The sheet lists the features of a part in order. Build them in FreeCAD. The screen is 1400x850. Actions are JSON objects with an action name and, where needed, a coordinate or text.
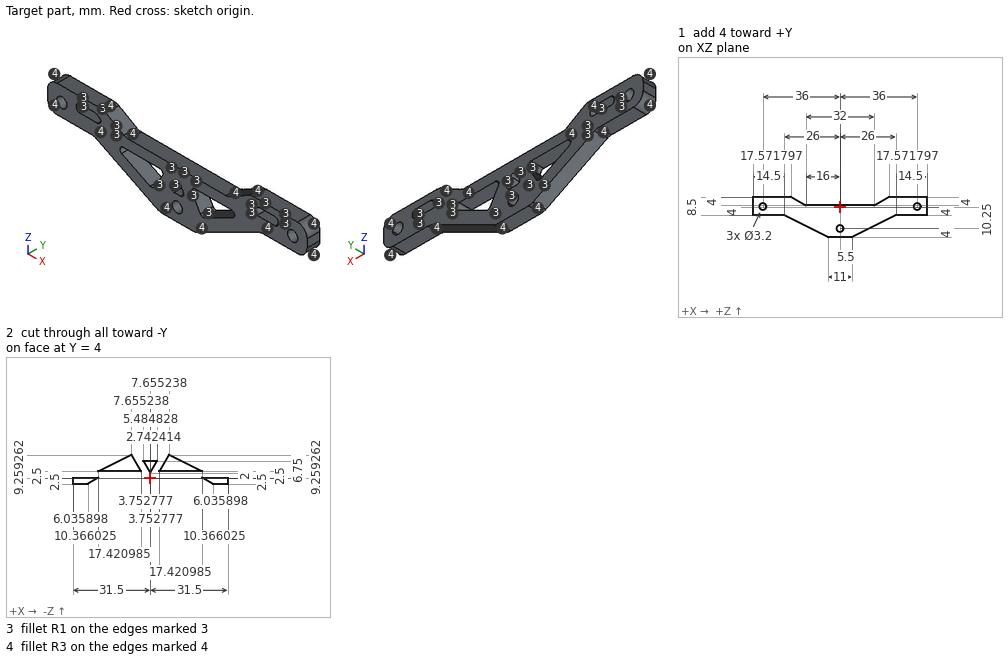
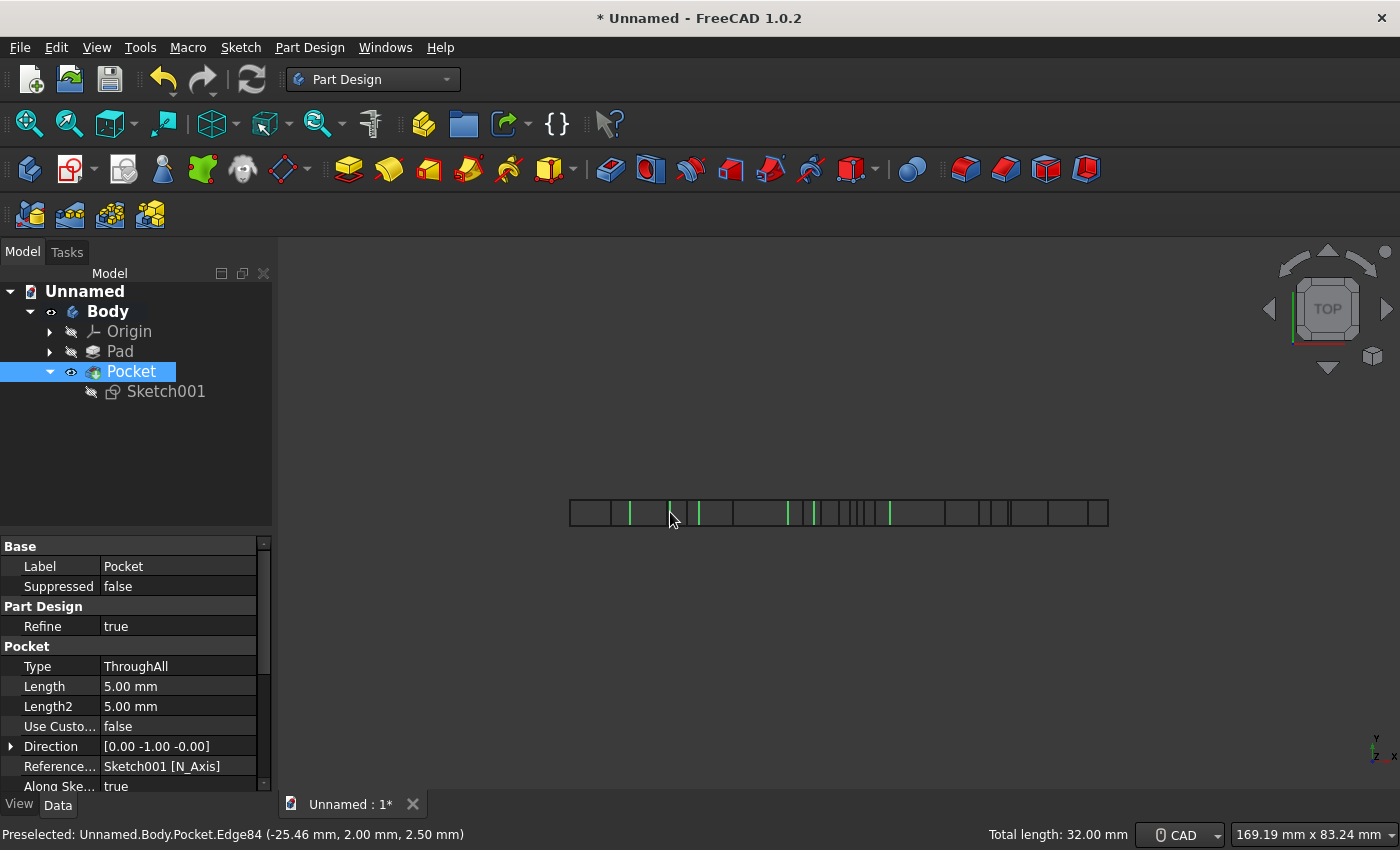
{"action": "left_click", "coordinate": [1008, 512], "text": "ctrl"}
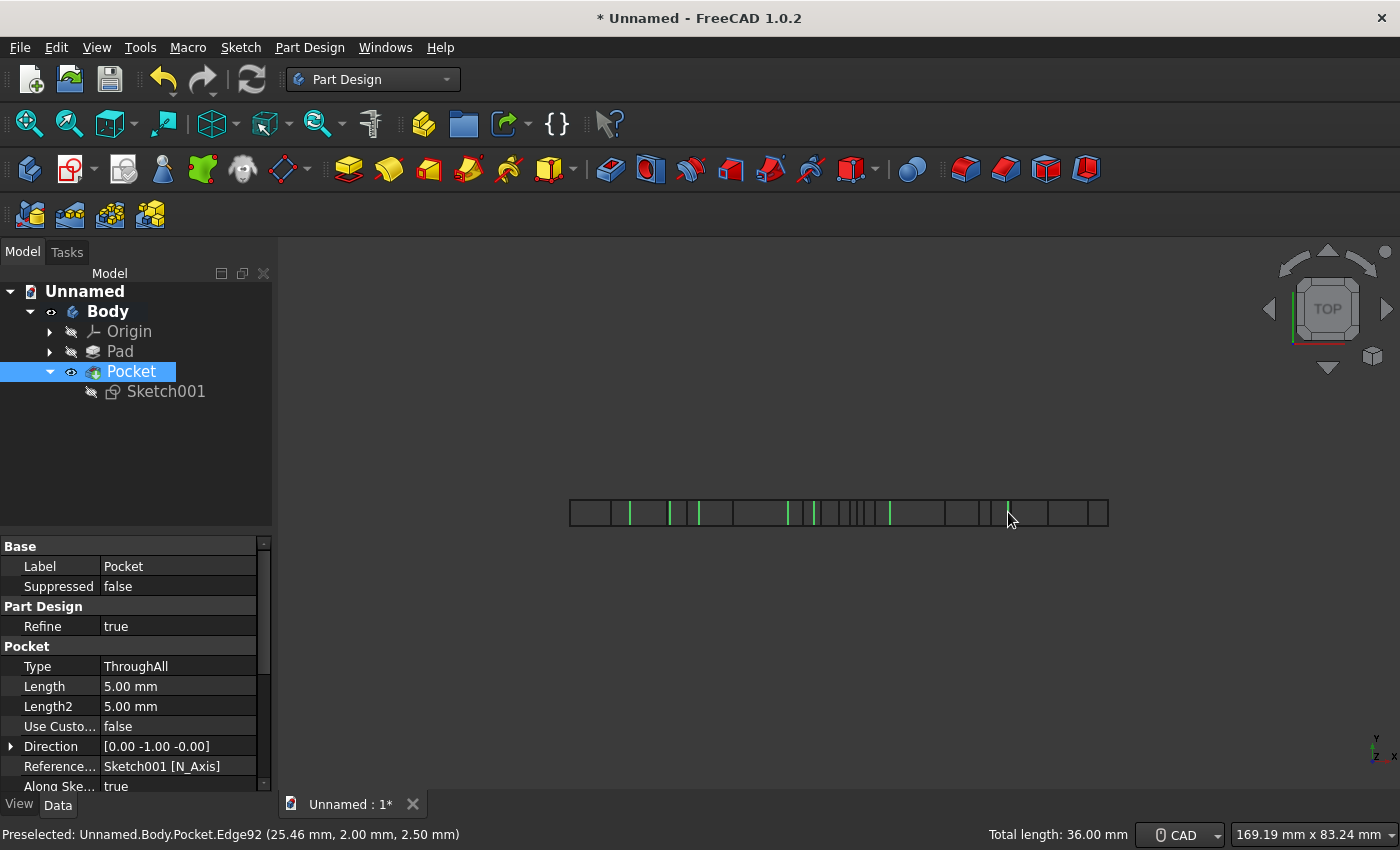
{"action": "left_click", "coordinate": [979, 512], "text": "ctrl"}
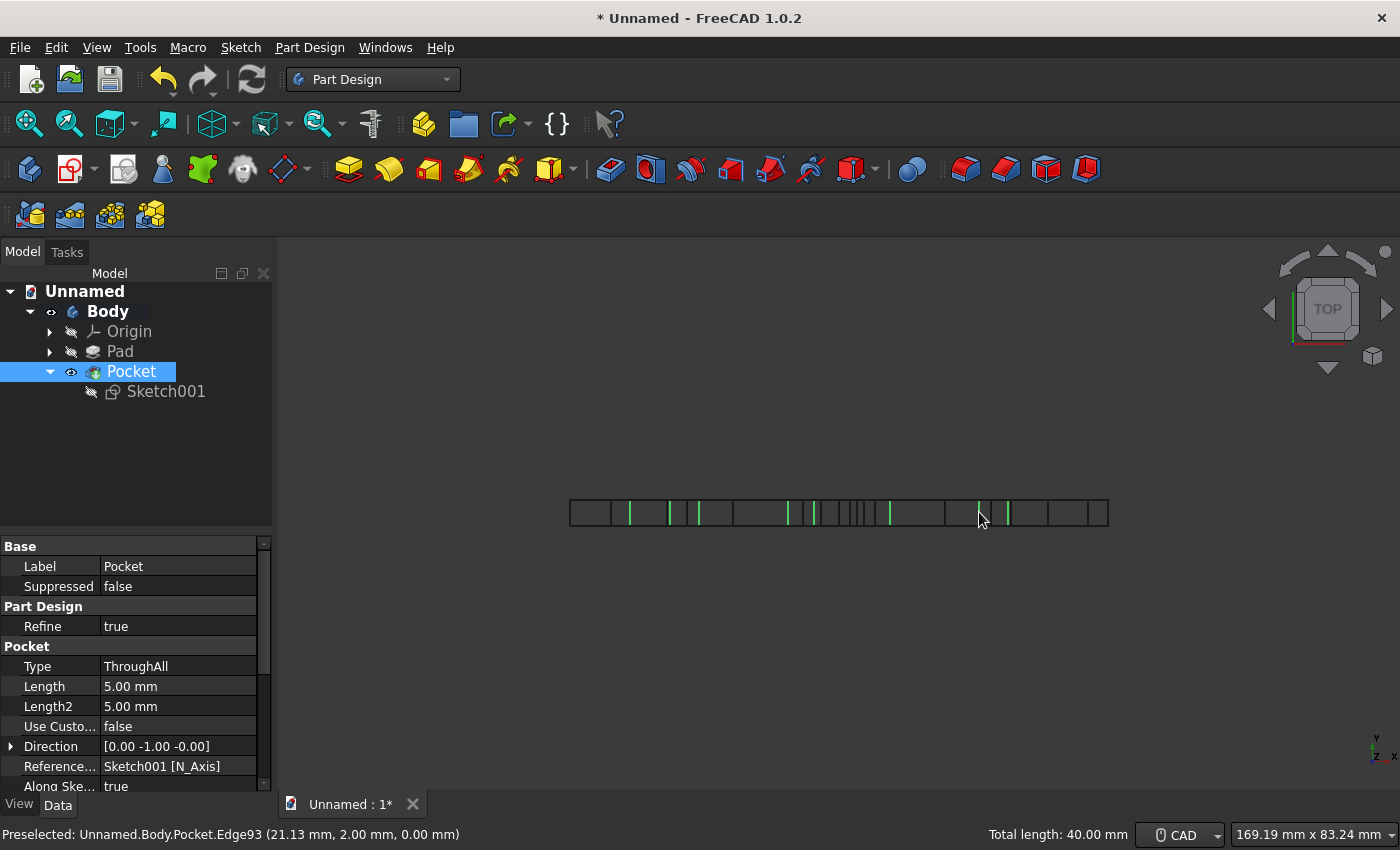
{"action": "left_click", "coordinate": [1048, 512], "text": "ctrl"}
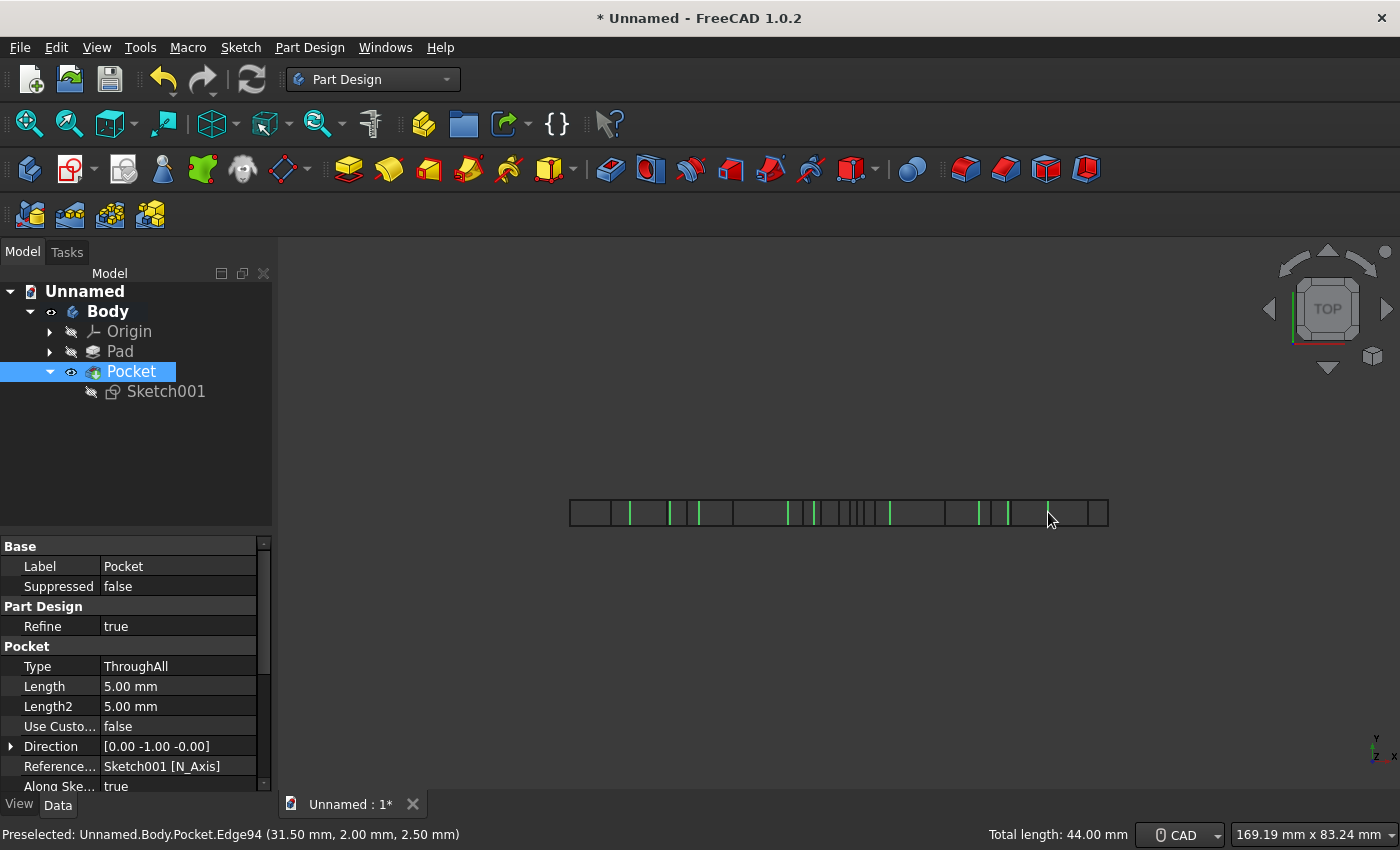
{"action": "left_click", "coordinate": [864, 512], "text": "ctrl"}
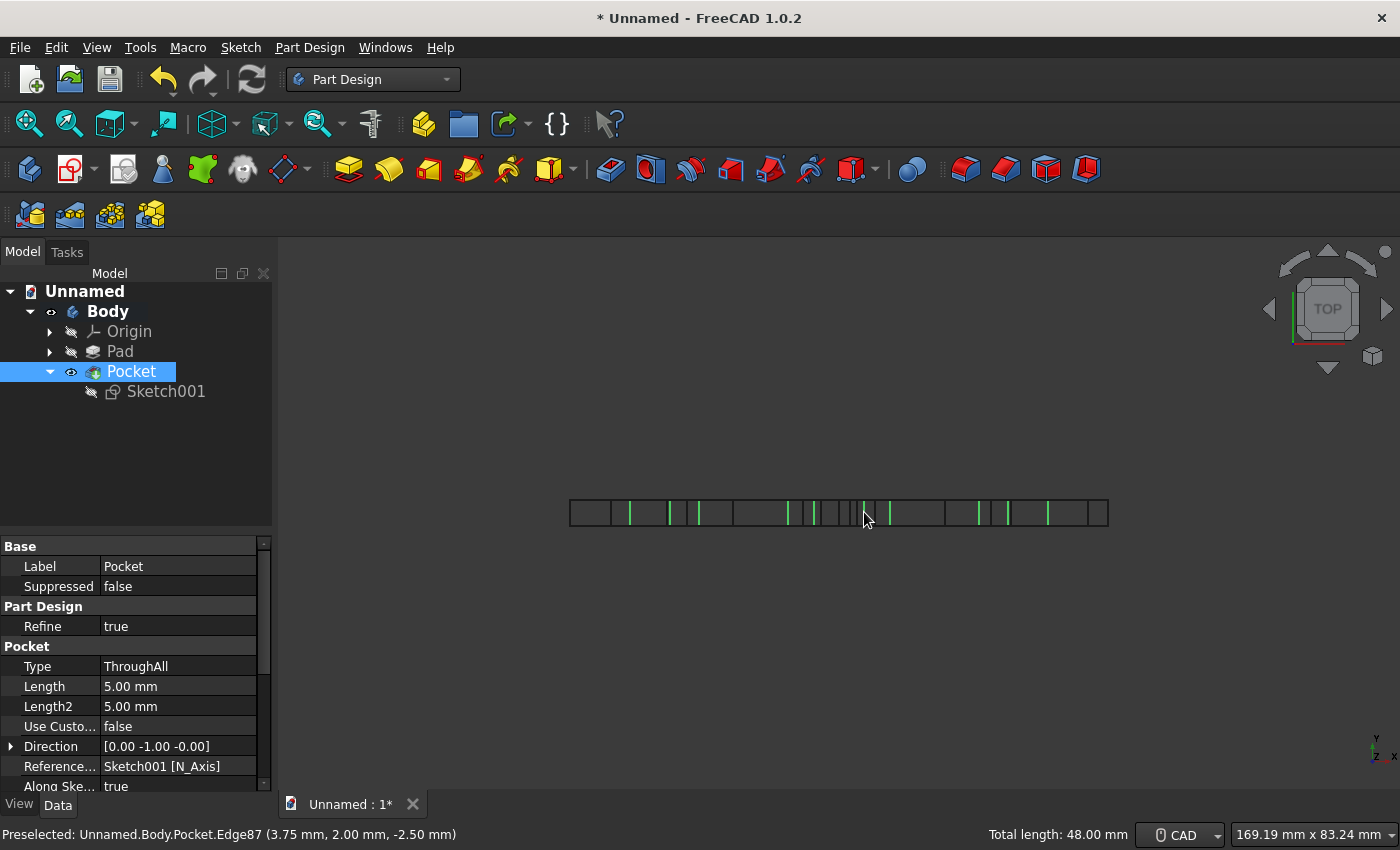
{"action": "left_click", "coordinate": [821, 512], "text": "ctrl"}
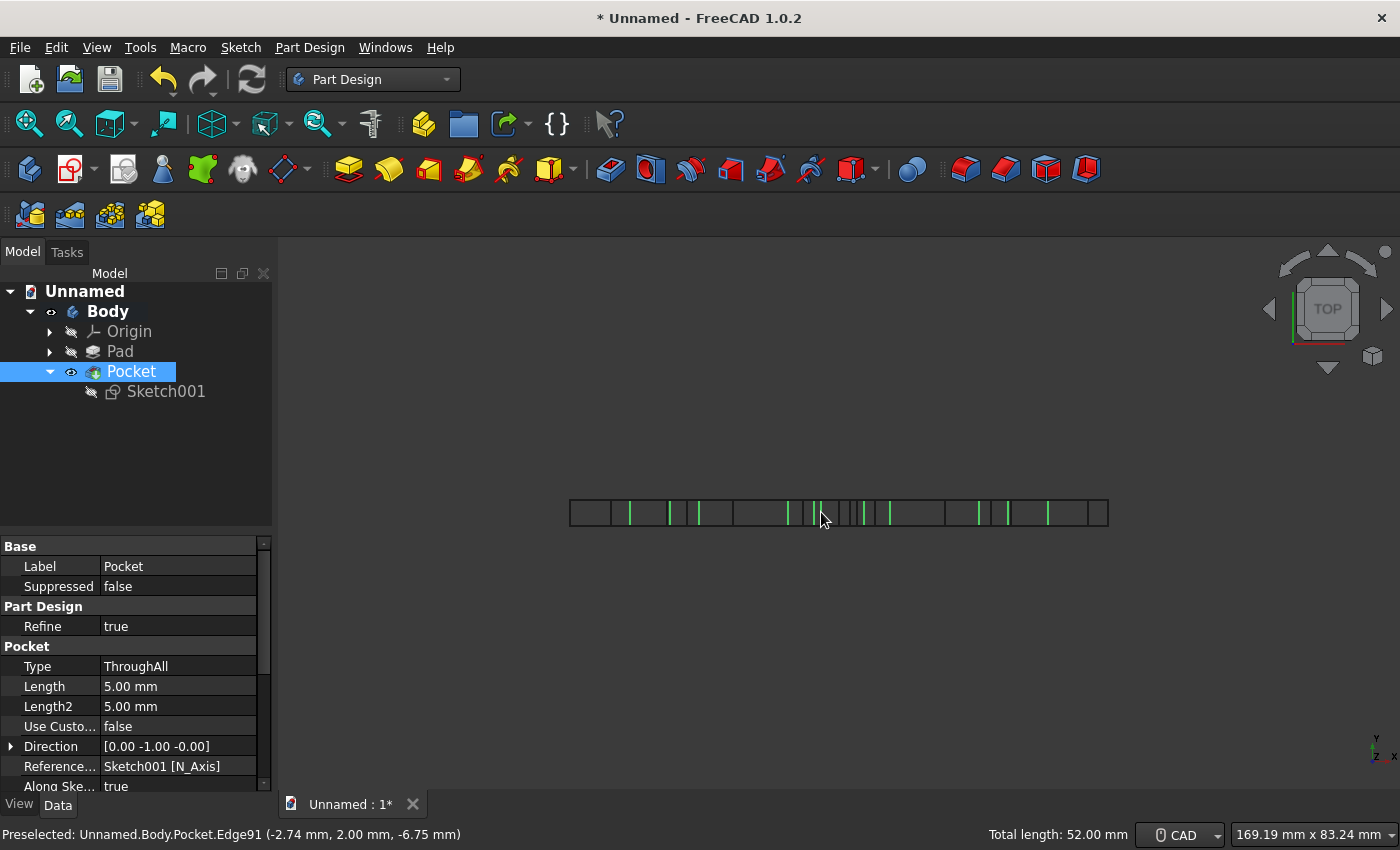
{"action": "left_click", "coordinate": [857, 512], "text": "ctrl"}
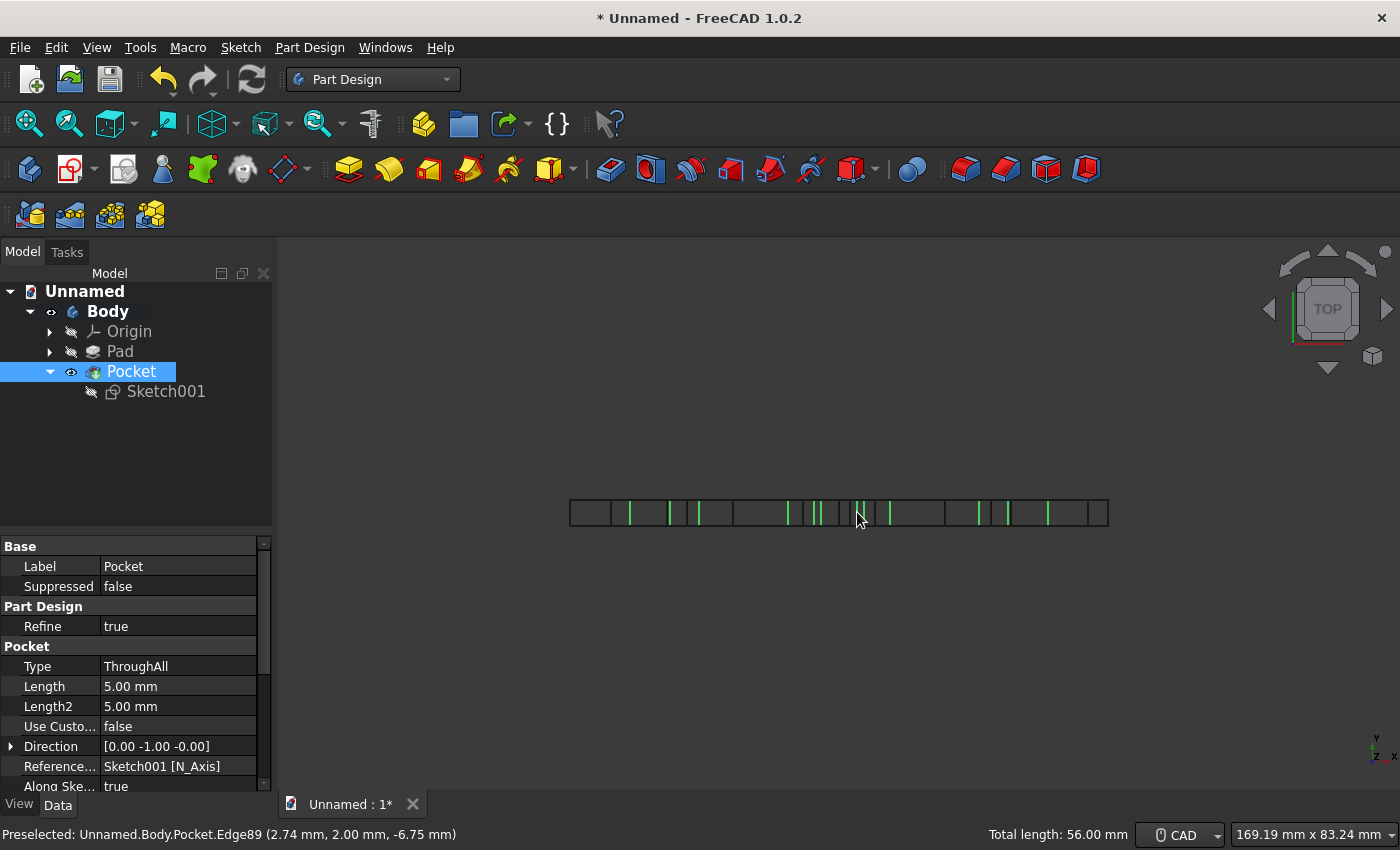
{"action": "left_click", "coordinate": [839, 512], "text": "ctrl"}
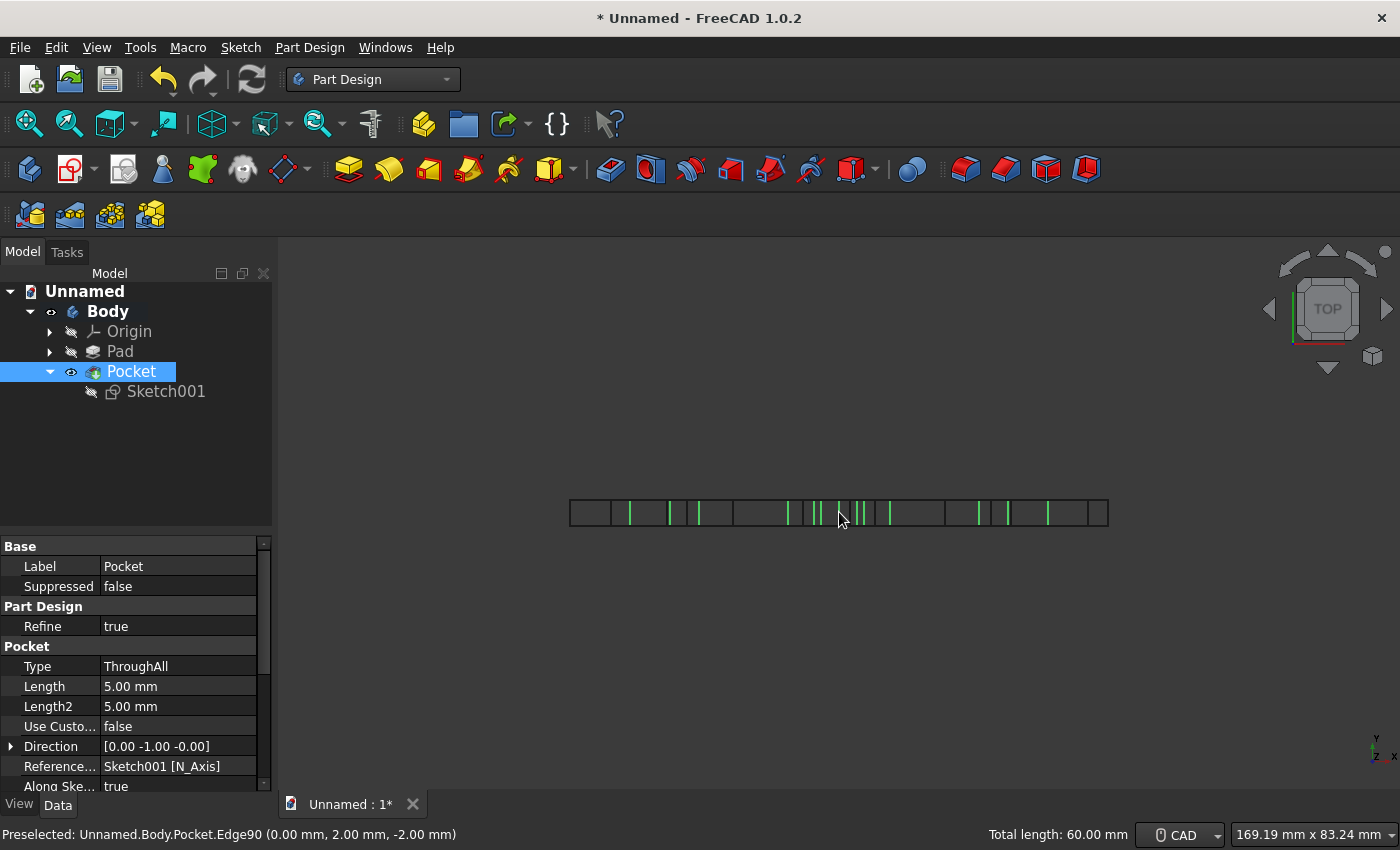
{"action": "key", "text": "1"}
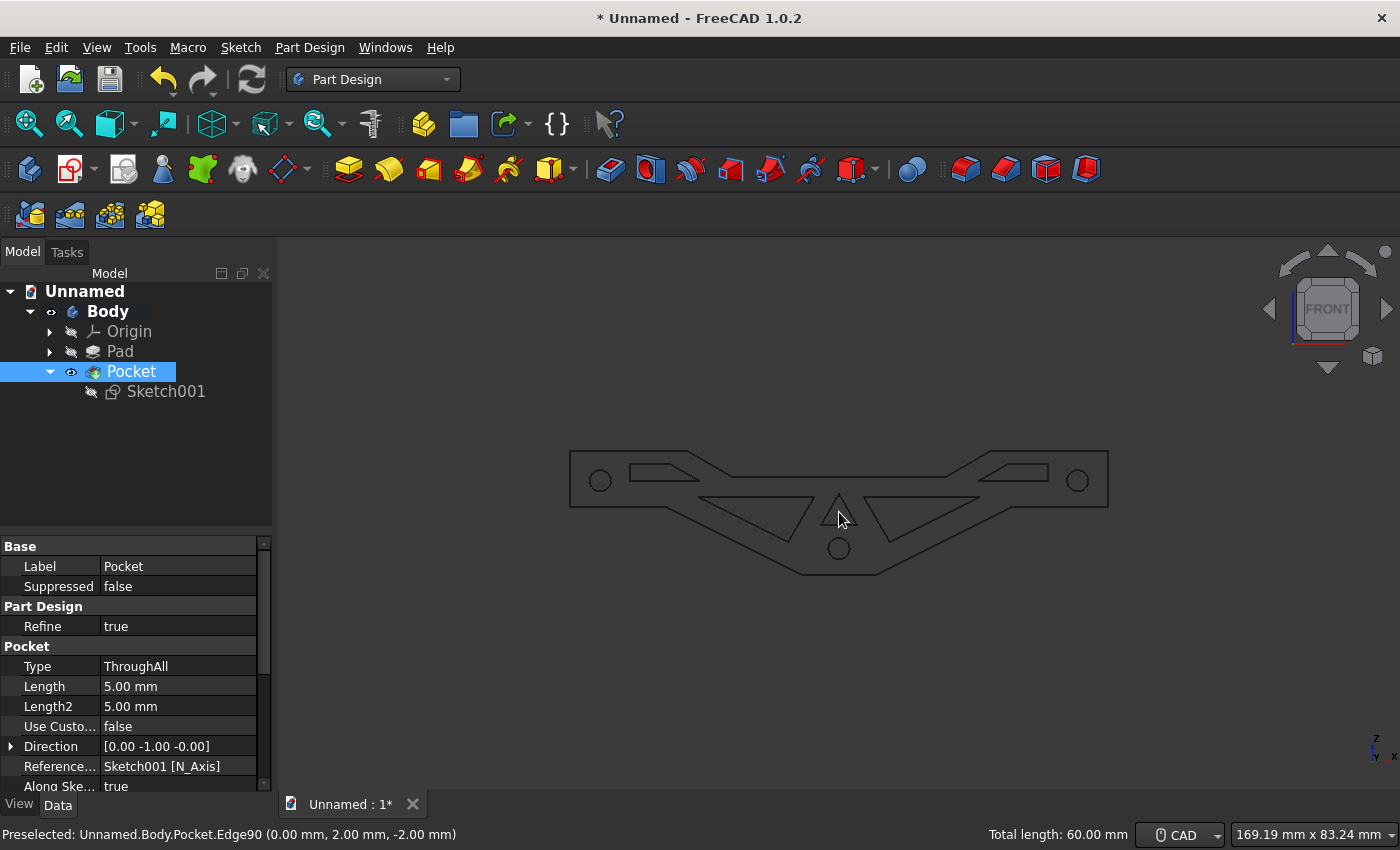
{"action": "key", "text": "3"}